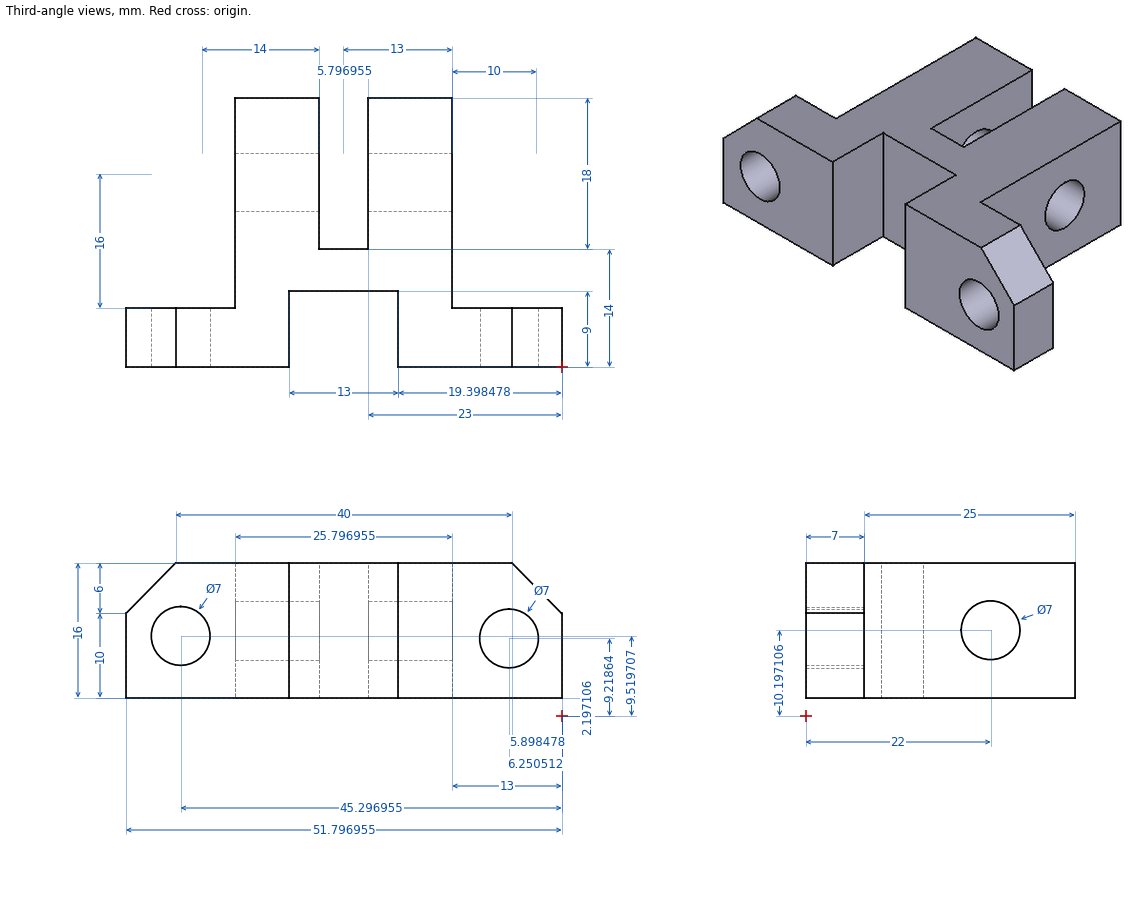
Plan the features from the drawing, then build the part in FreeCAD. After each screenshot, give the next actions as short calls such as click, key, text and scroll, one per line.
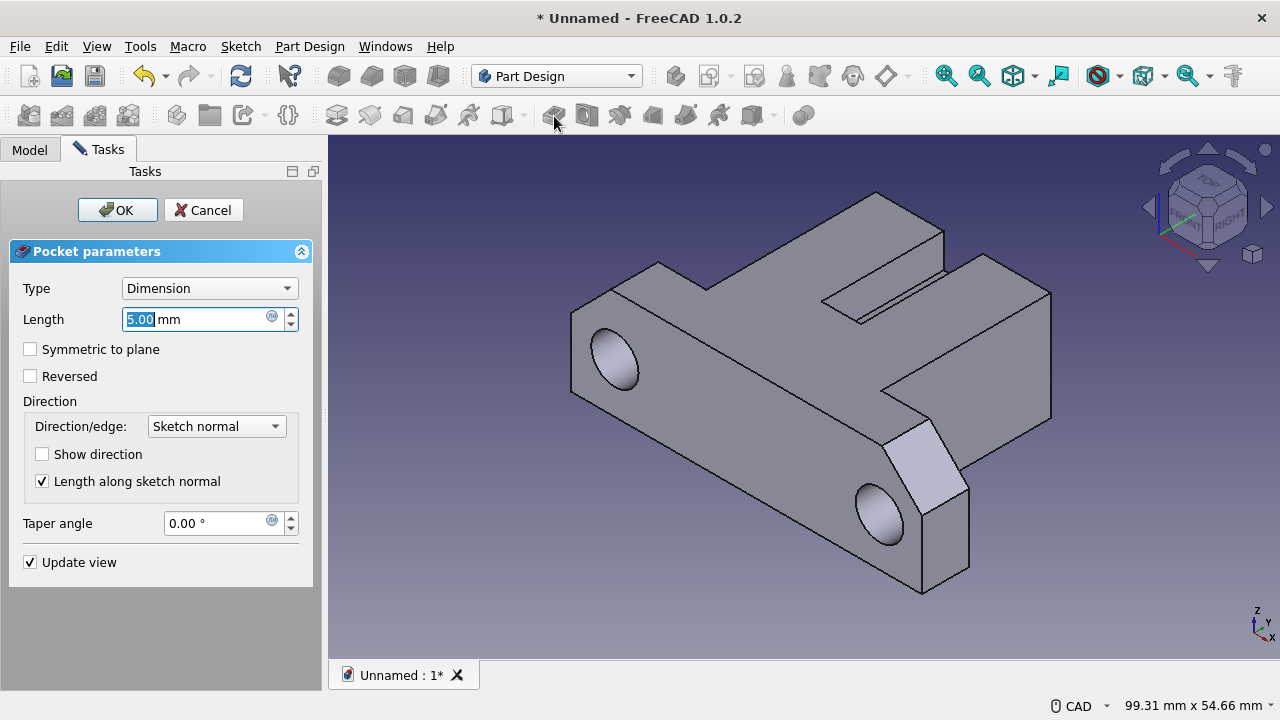
click(210, 288)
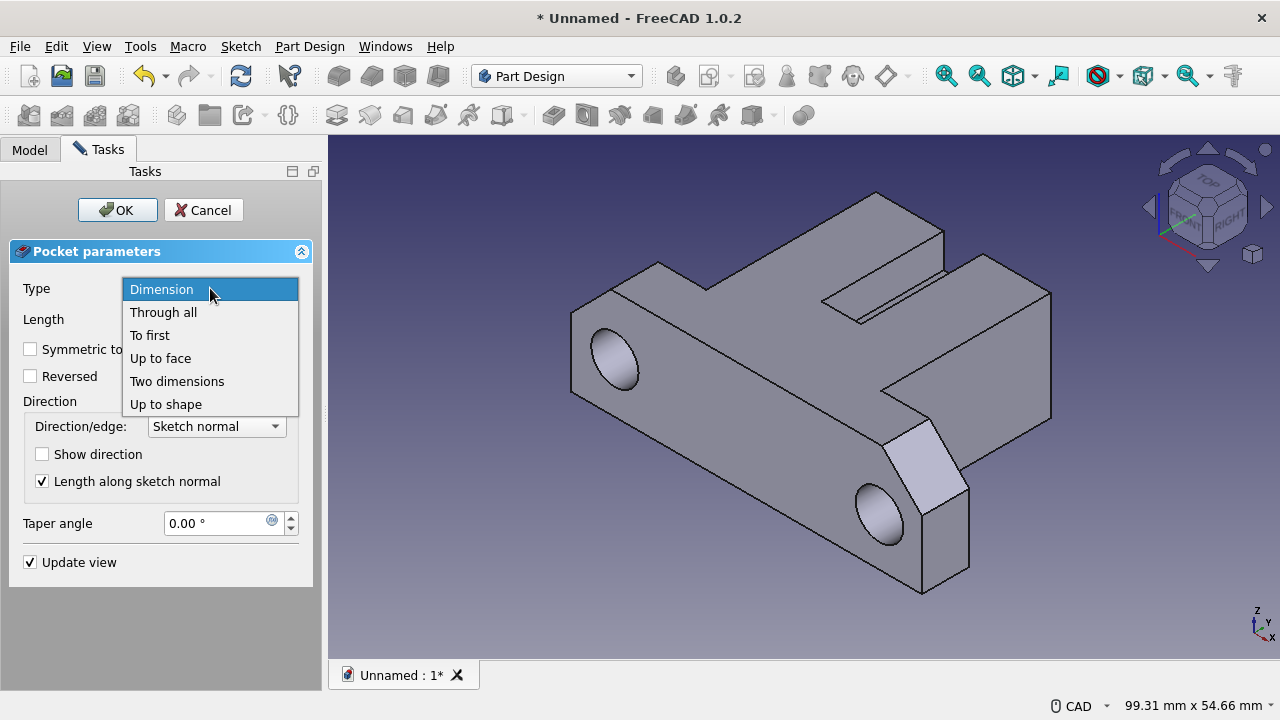
click(208, 382)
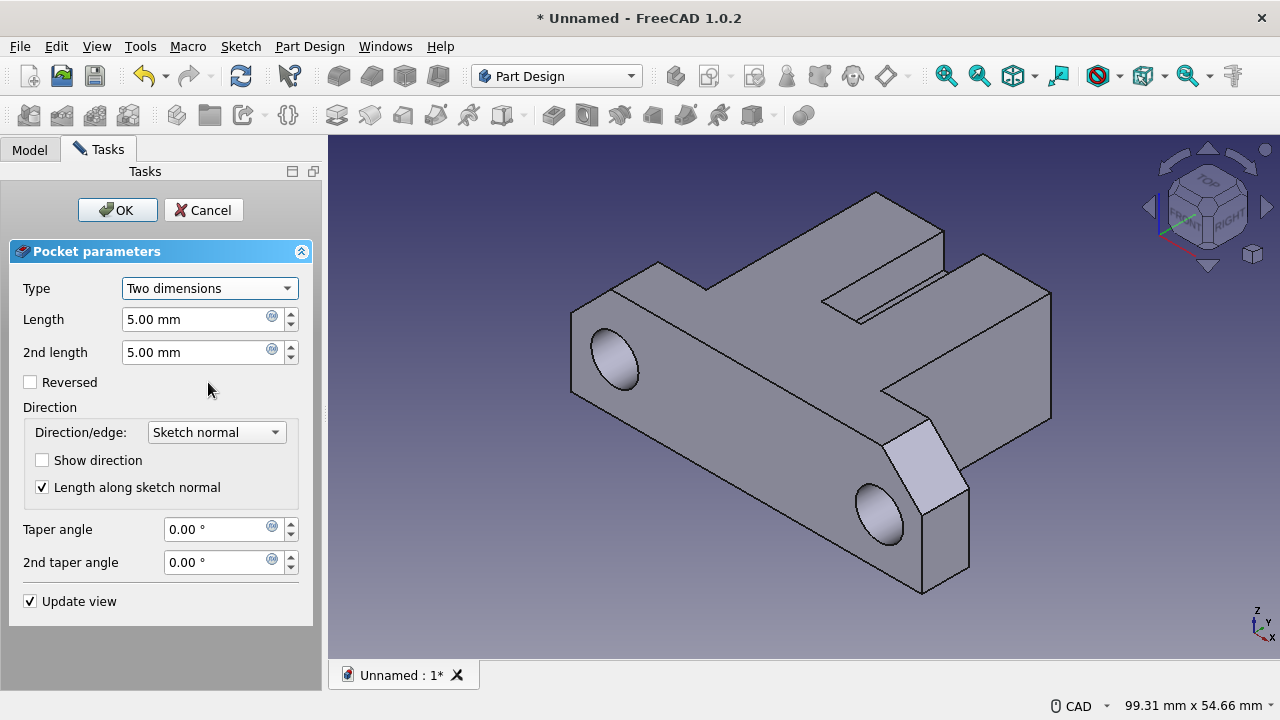
triple_click(204, 320)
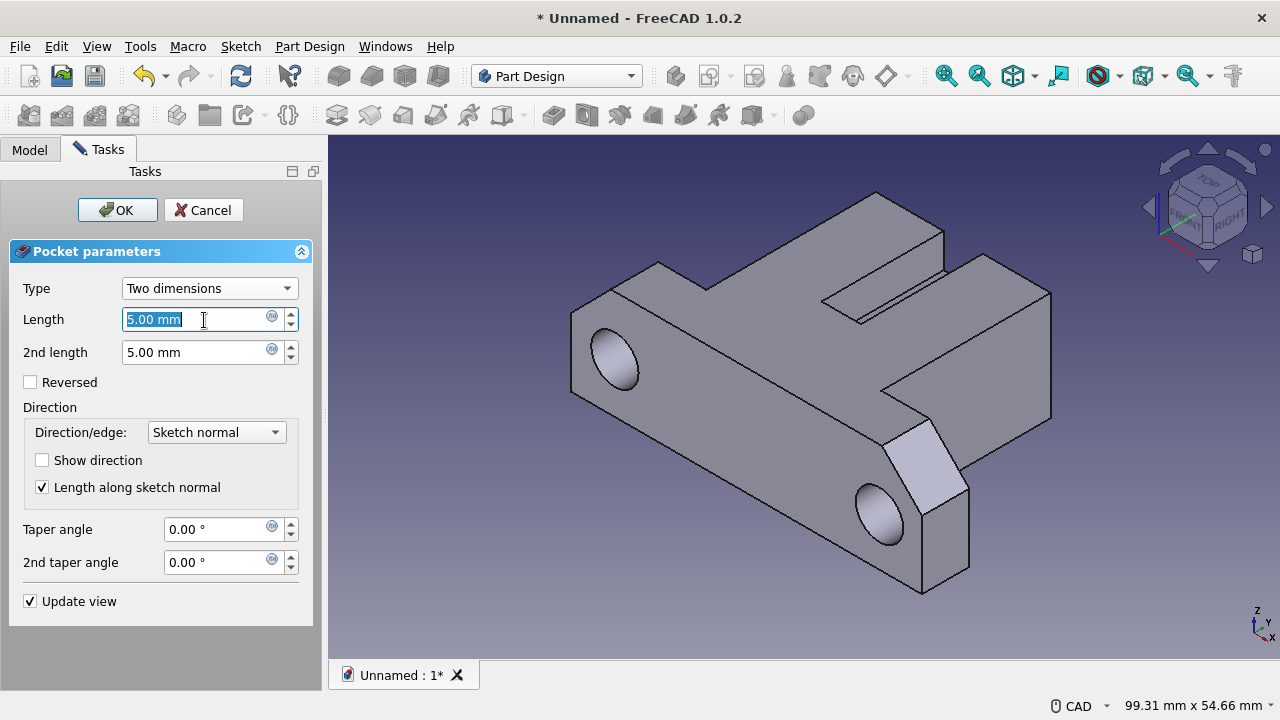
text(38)
key(Tab)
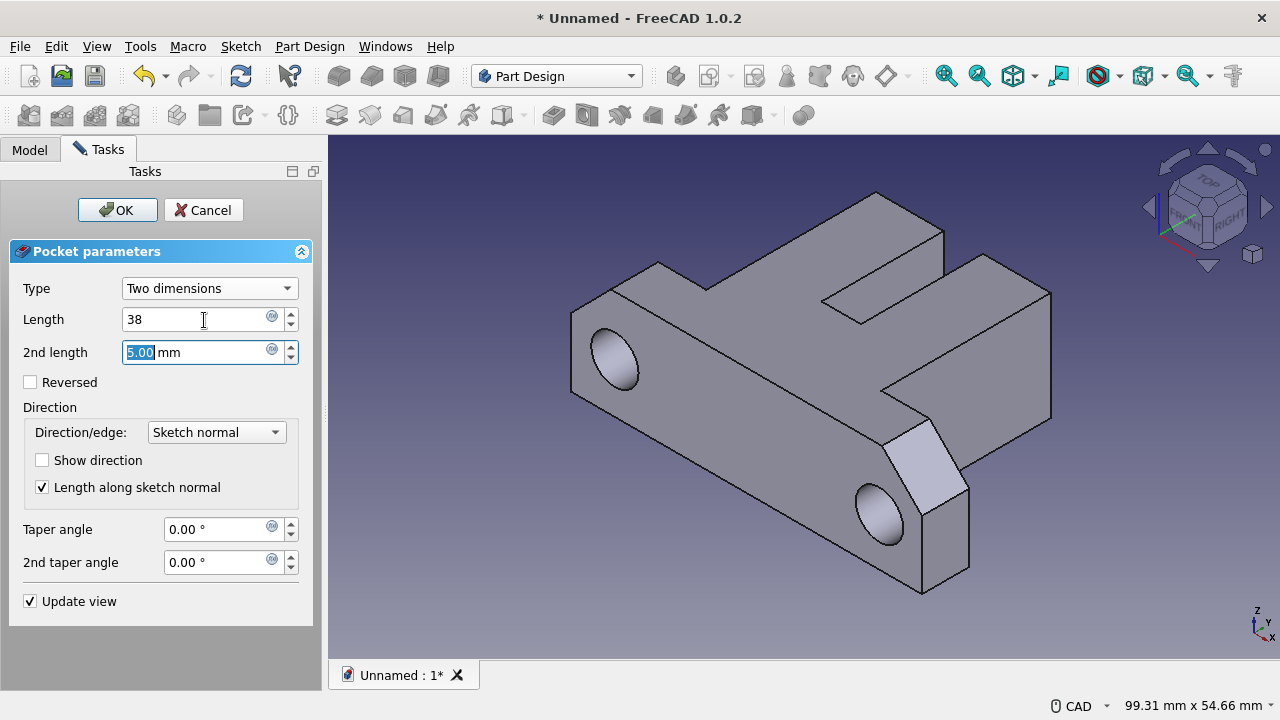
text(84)
key(Tab)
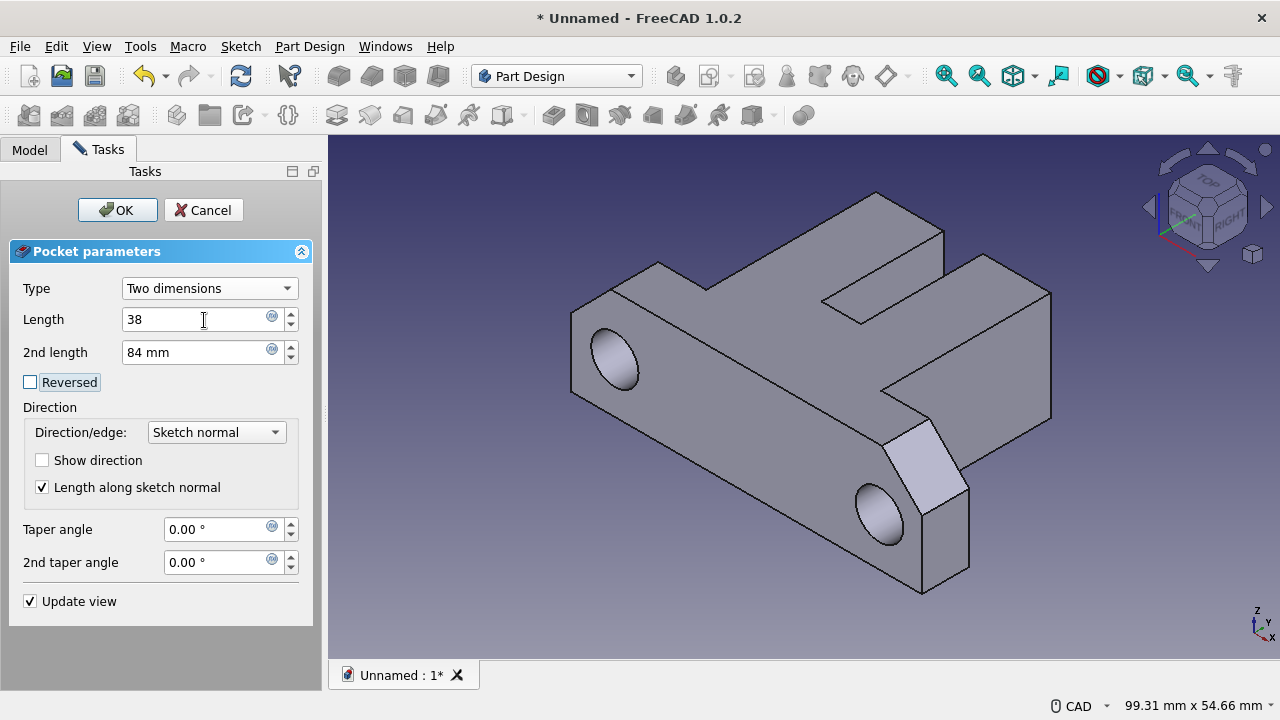
click(31, 382)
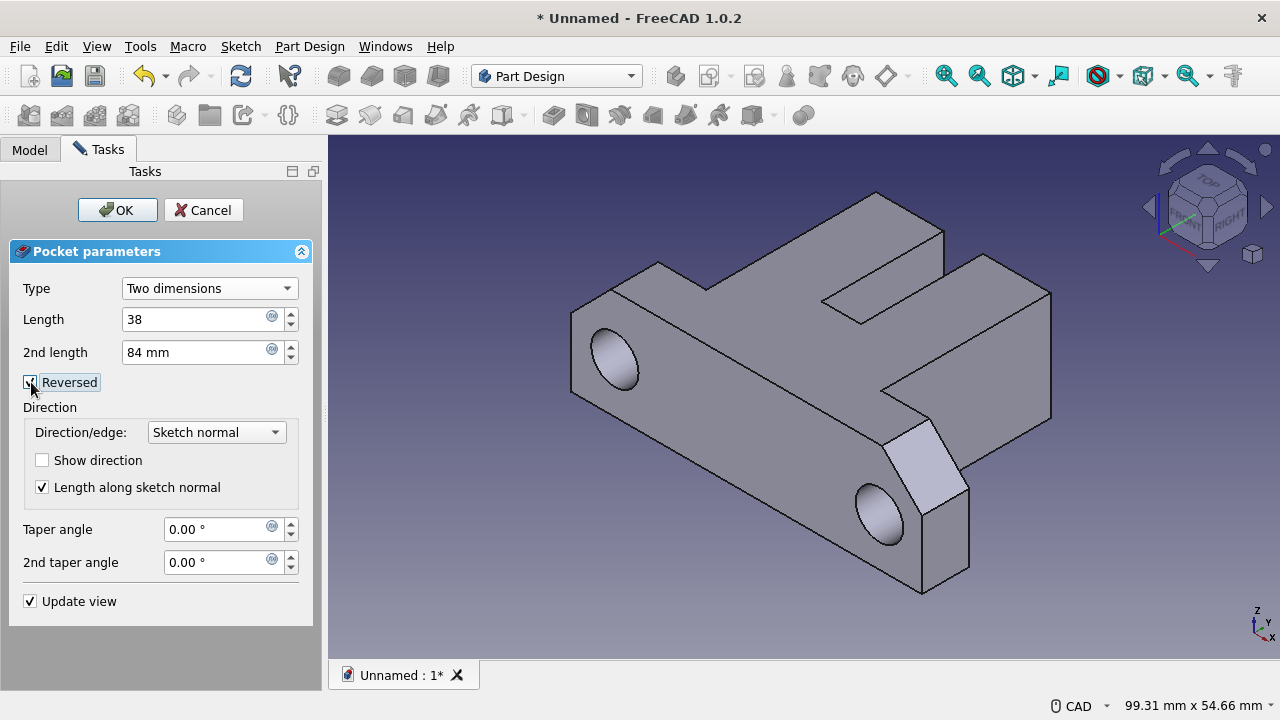
click(118, 210)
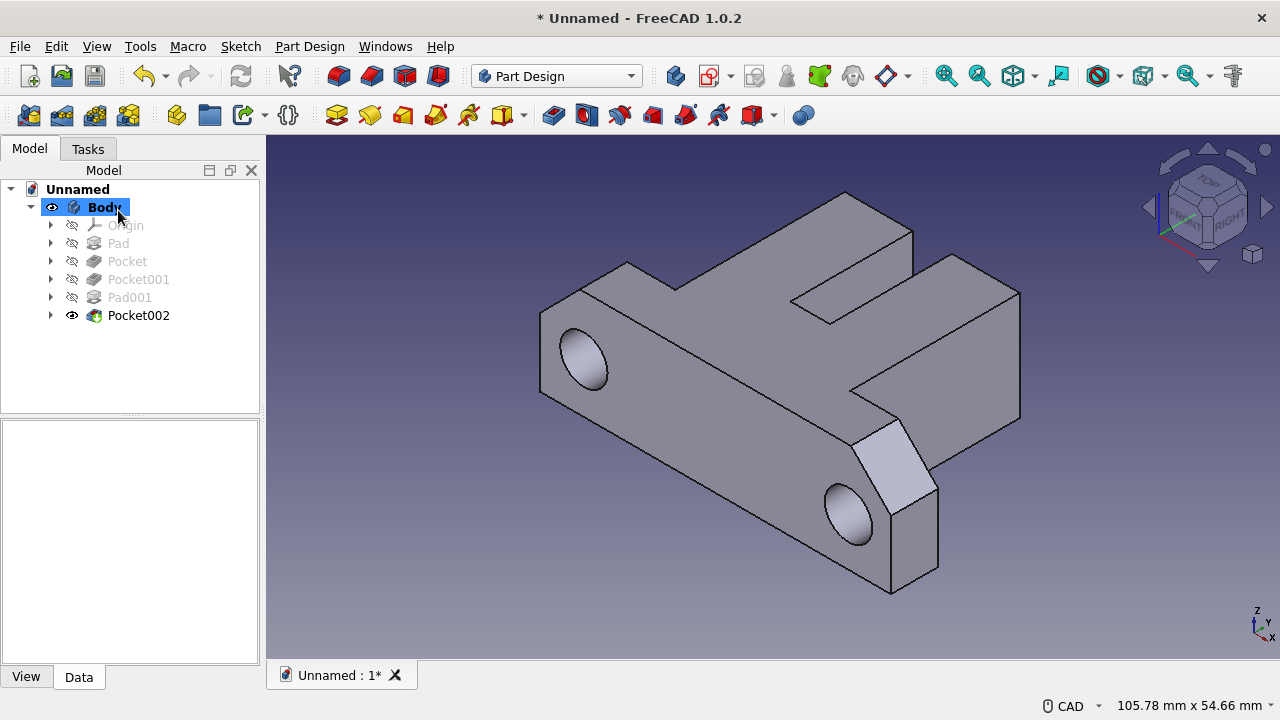
click(935, 403)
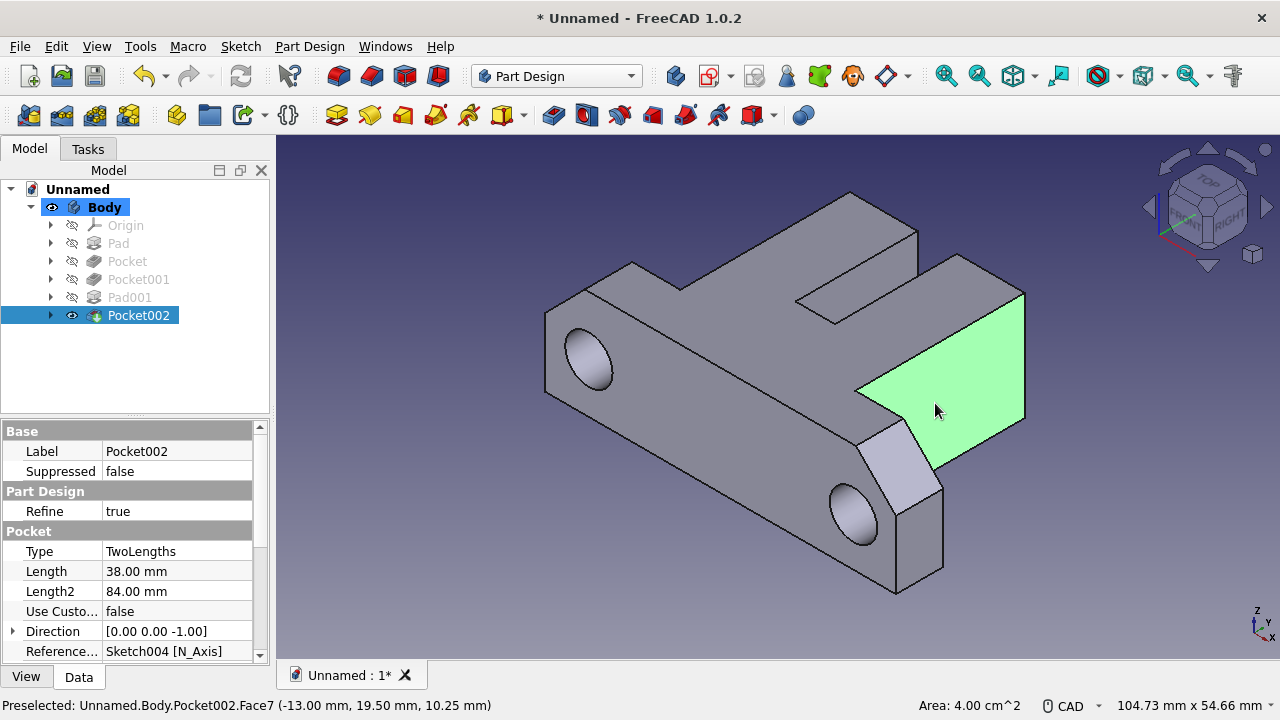
click(708, 76)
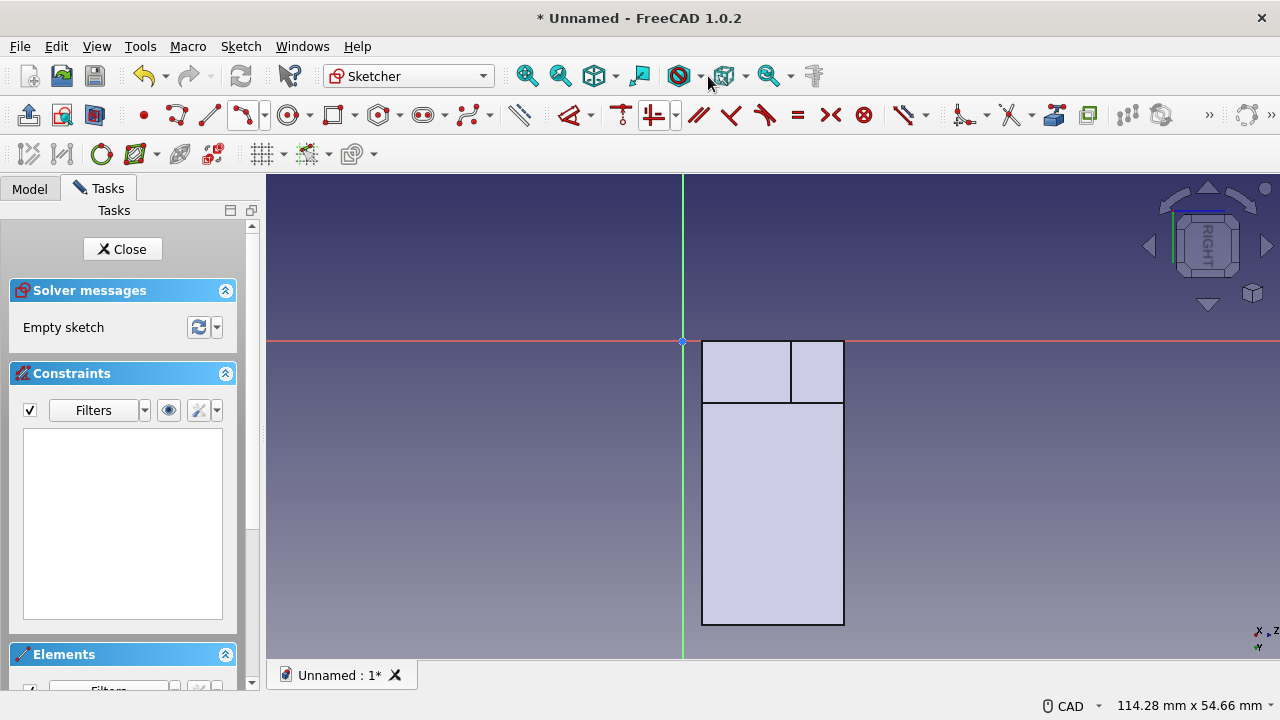
click(95, 116)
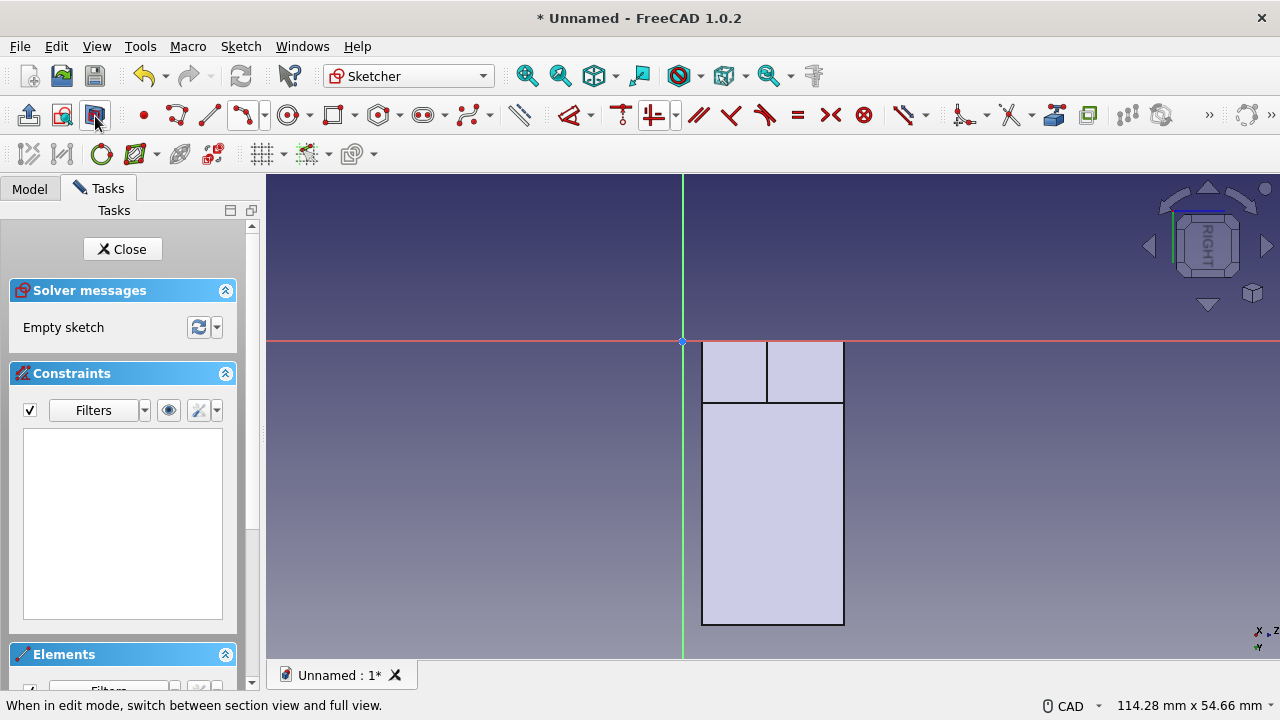
scroll(790, 567, up, 8)